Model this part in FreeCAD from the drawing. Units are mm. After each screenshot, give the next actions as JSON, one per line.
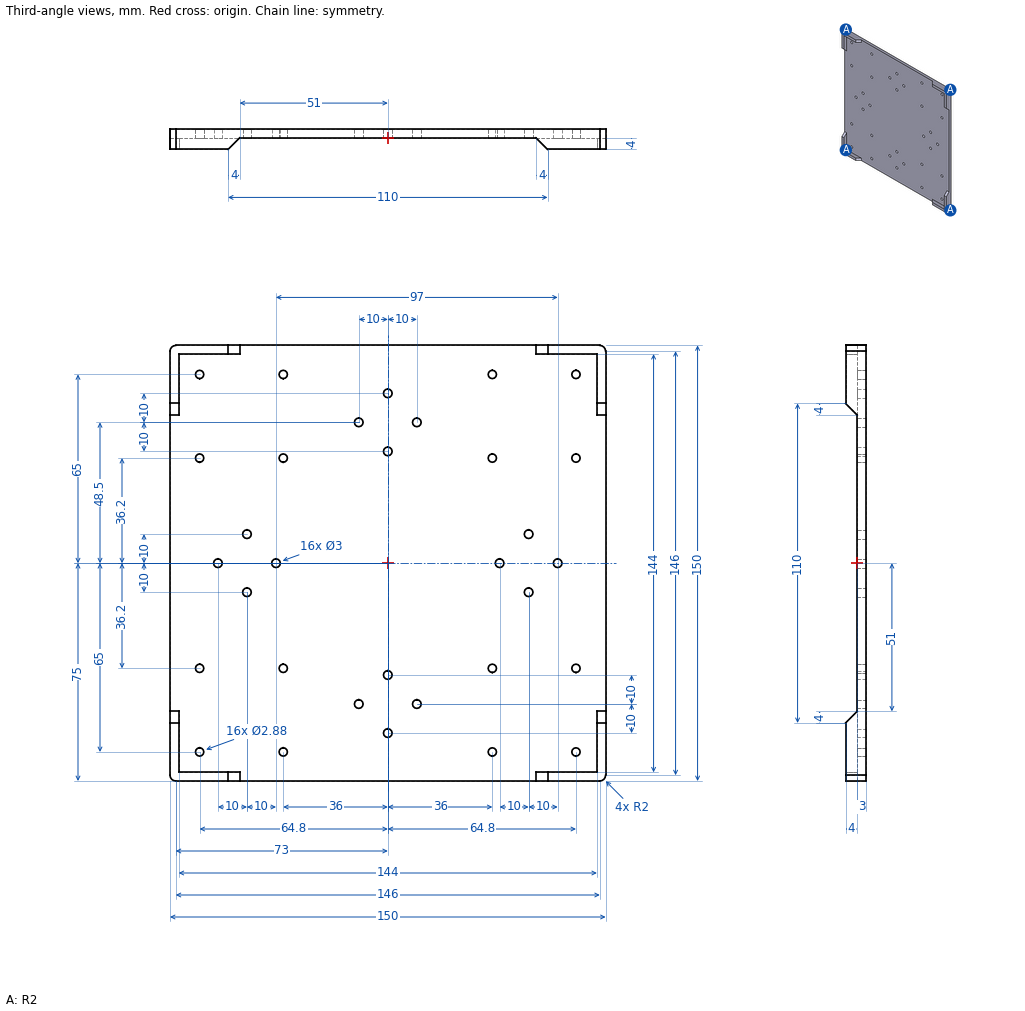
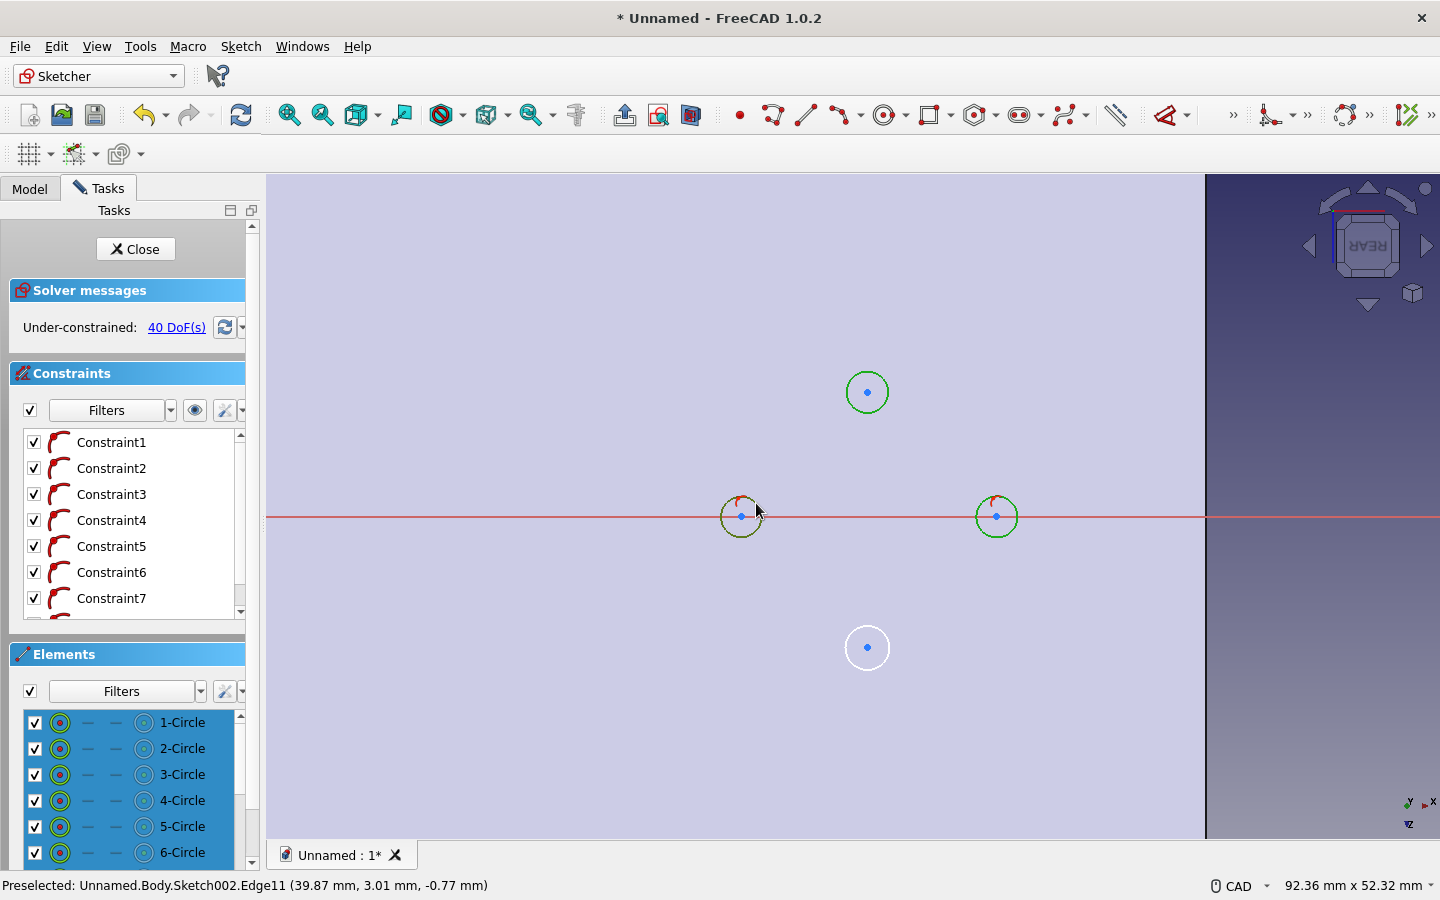
{"action": "scroll", "coordinate": [1014, 502], "scroll_direction": "down", "scroll_amount": 6}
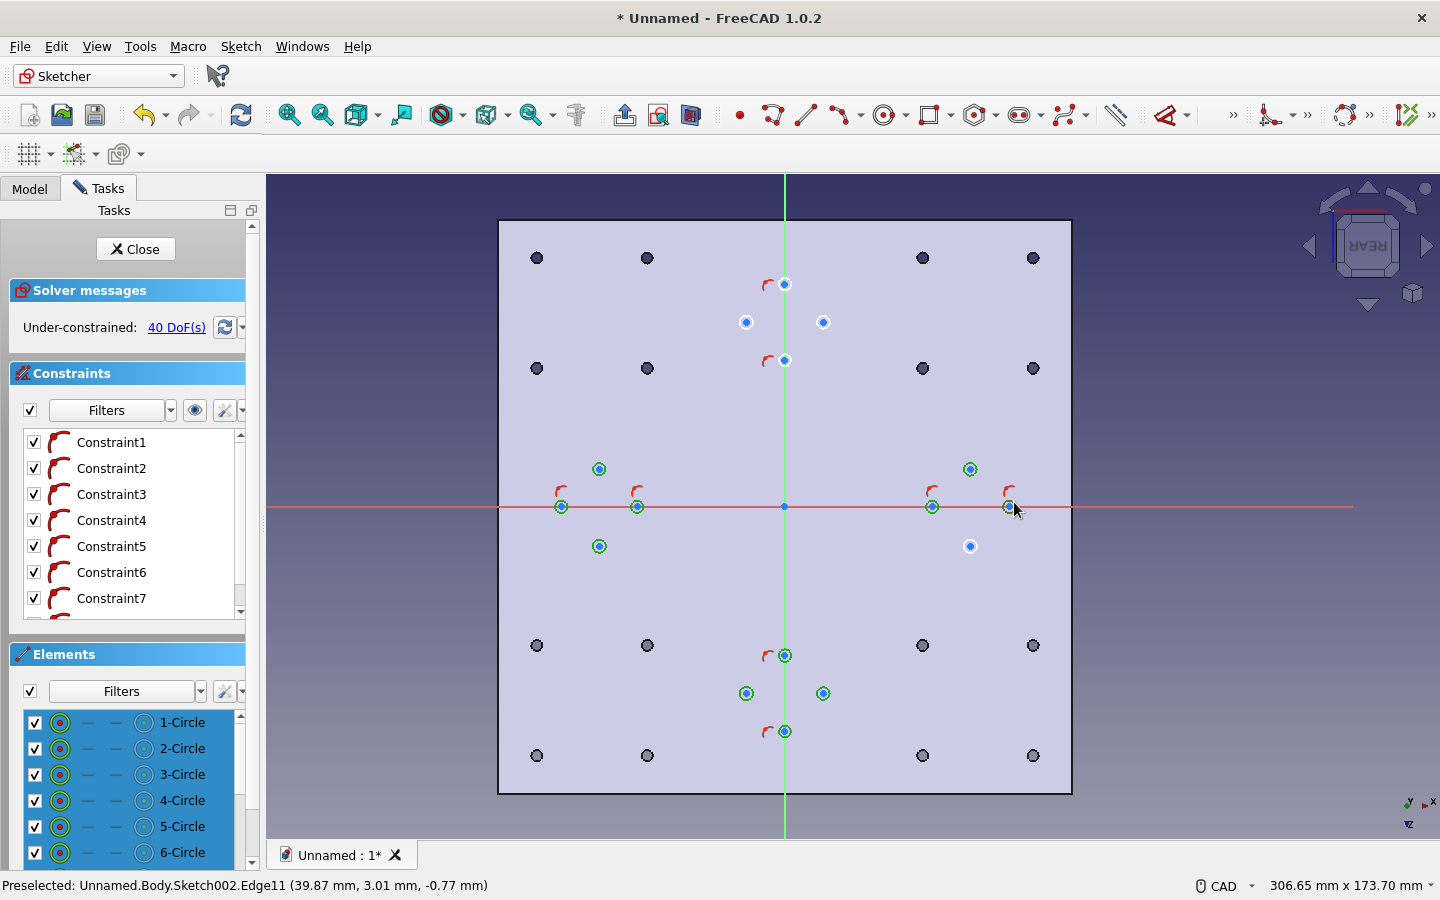
{"action": "scroll", "coordinate": [789, 356], "scroll_direction": "up", "scroll_amount": 7}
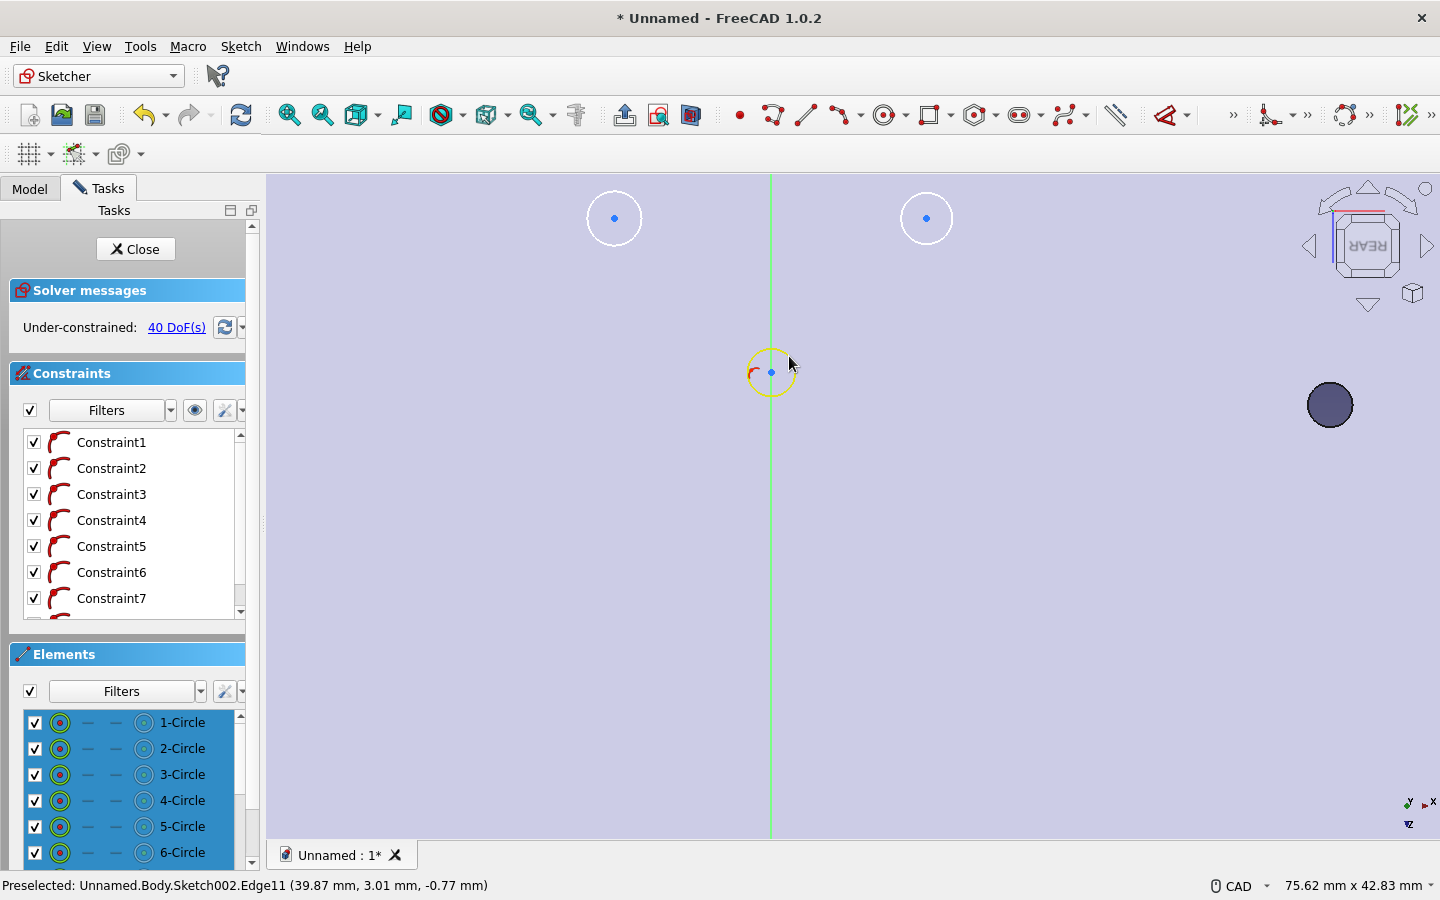
{"action": "left_click", "coordinate": [788, 356]}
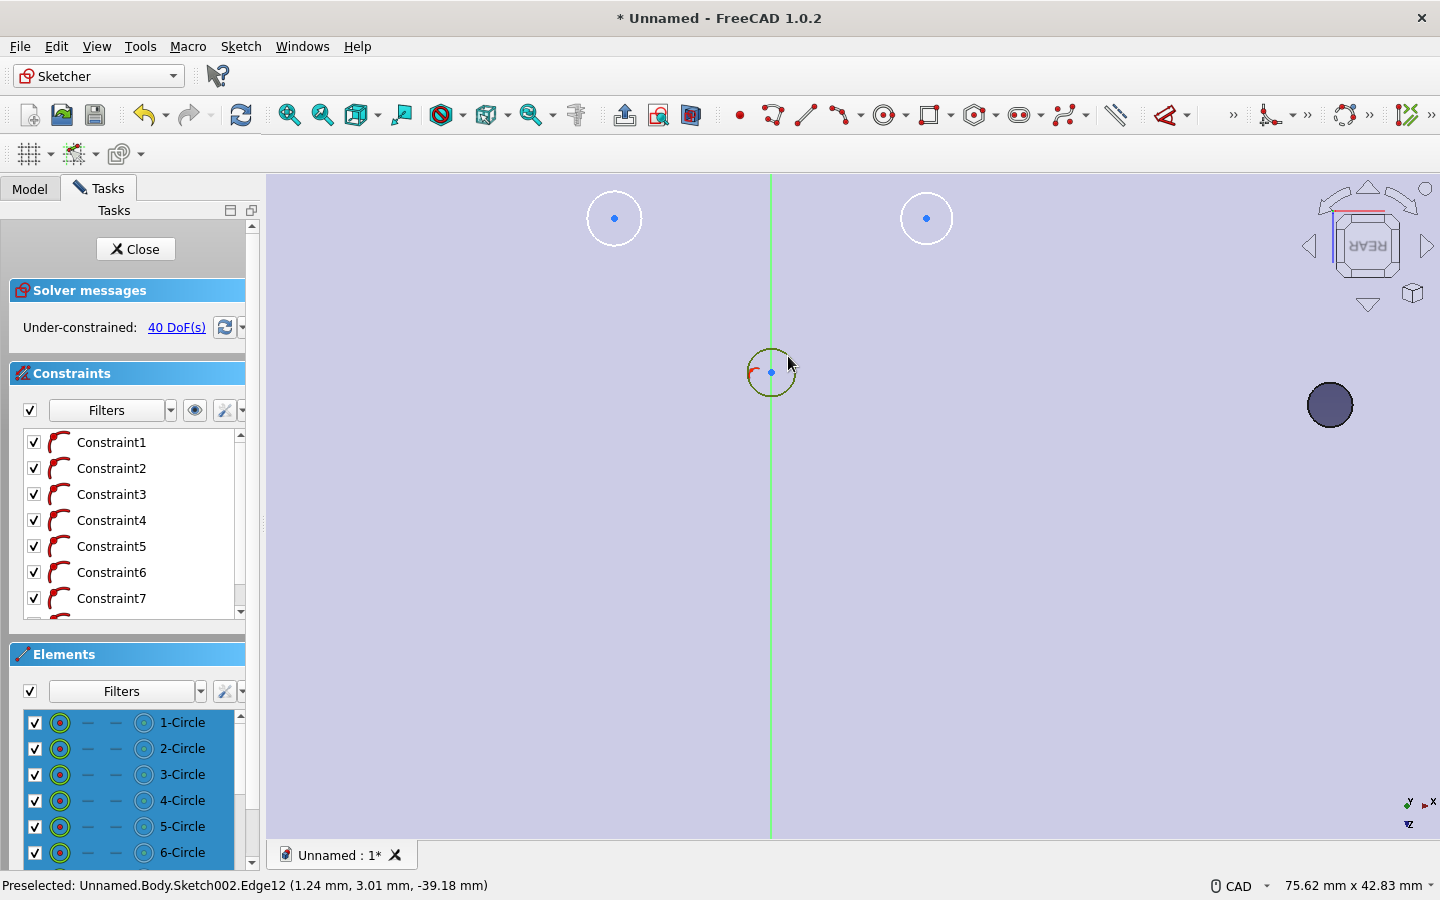
{"action": "left_click", "coordinate": [909, 237]}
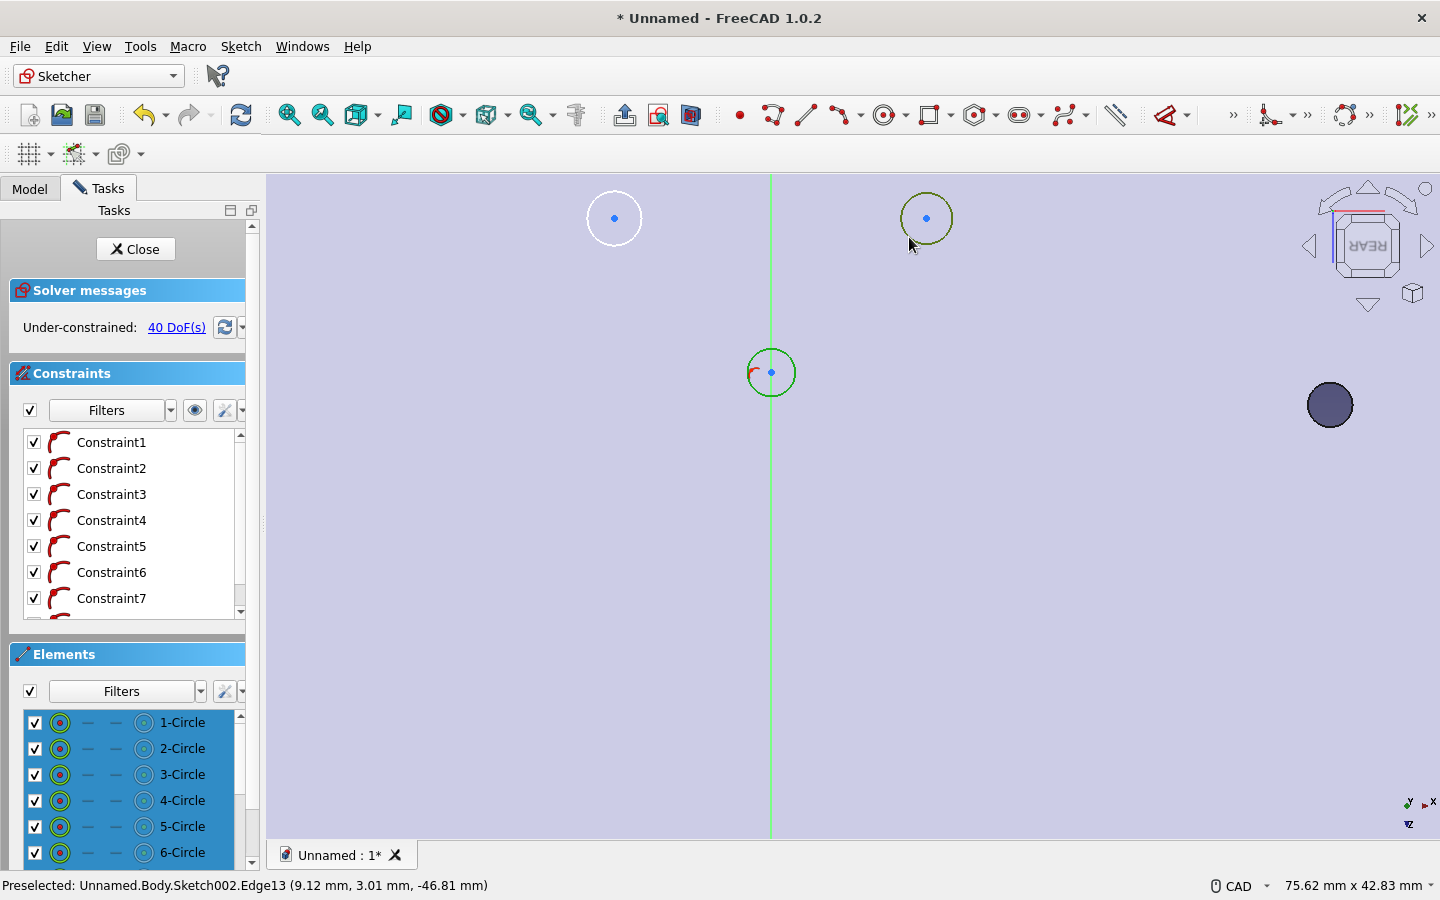
{"action": "scroll", "coordinate": [789, 356], "scroll_direction": "down", "scroll_amount": 7}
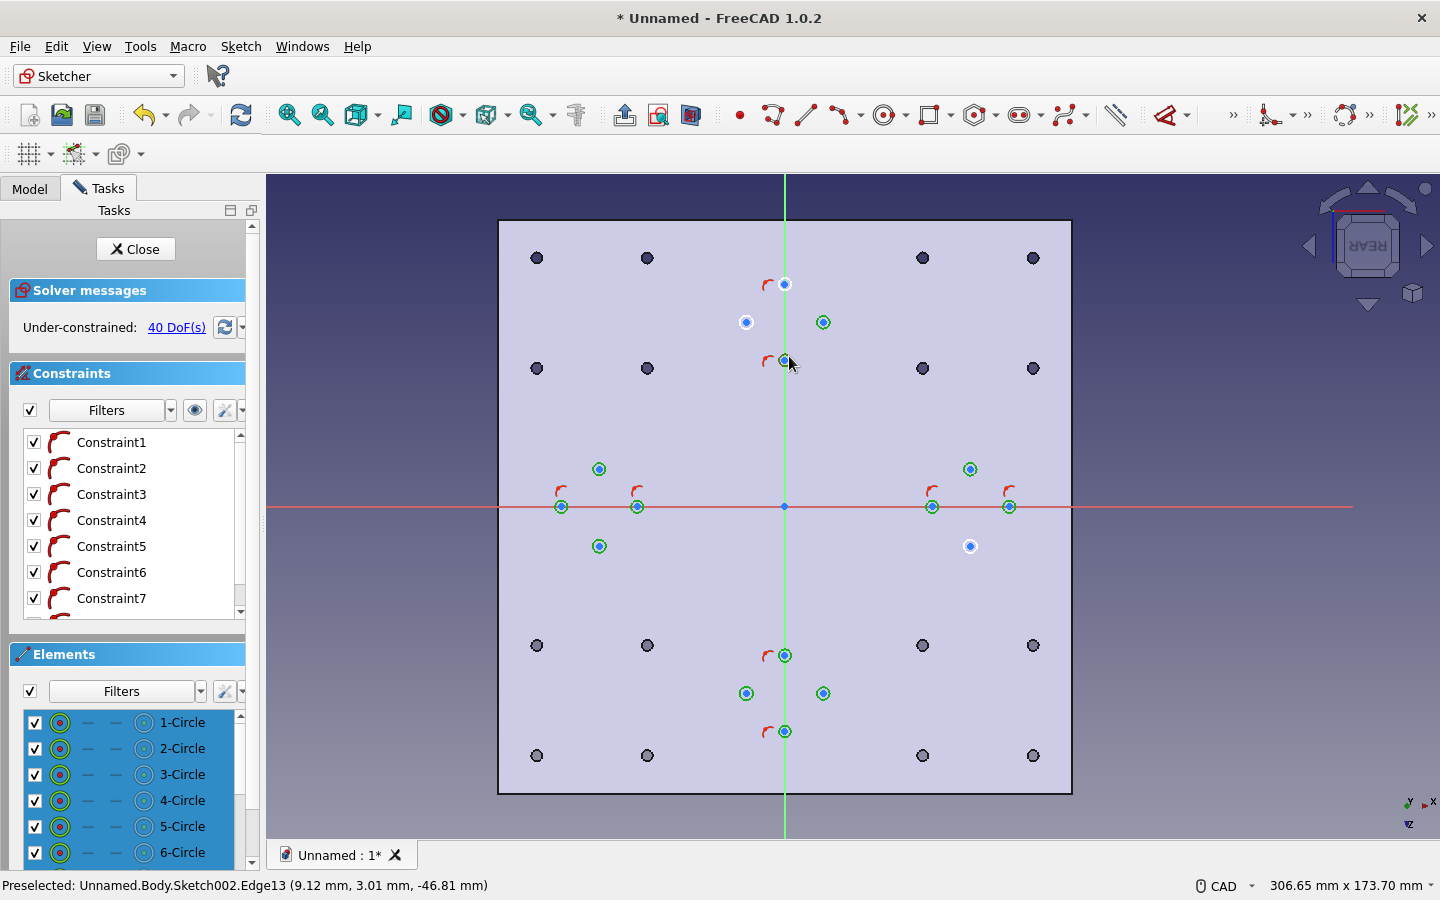
{"action": "scroll", "coordinate": [789, 280], "scroll_direction": "up", "scroll_amount": 6}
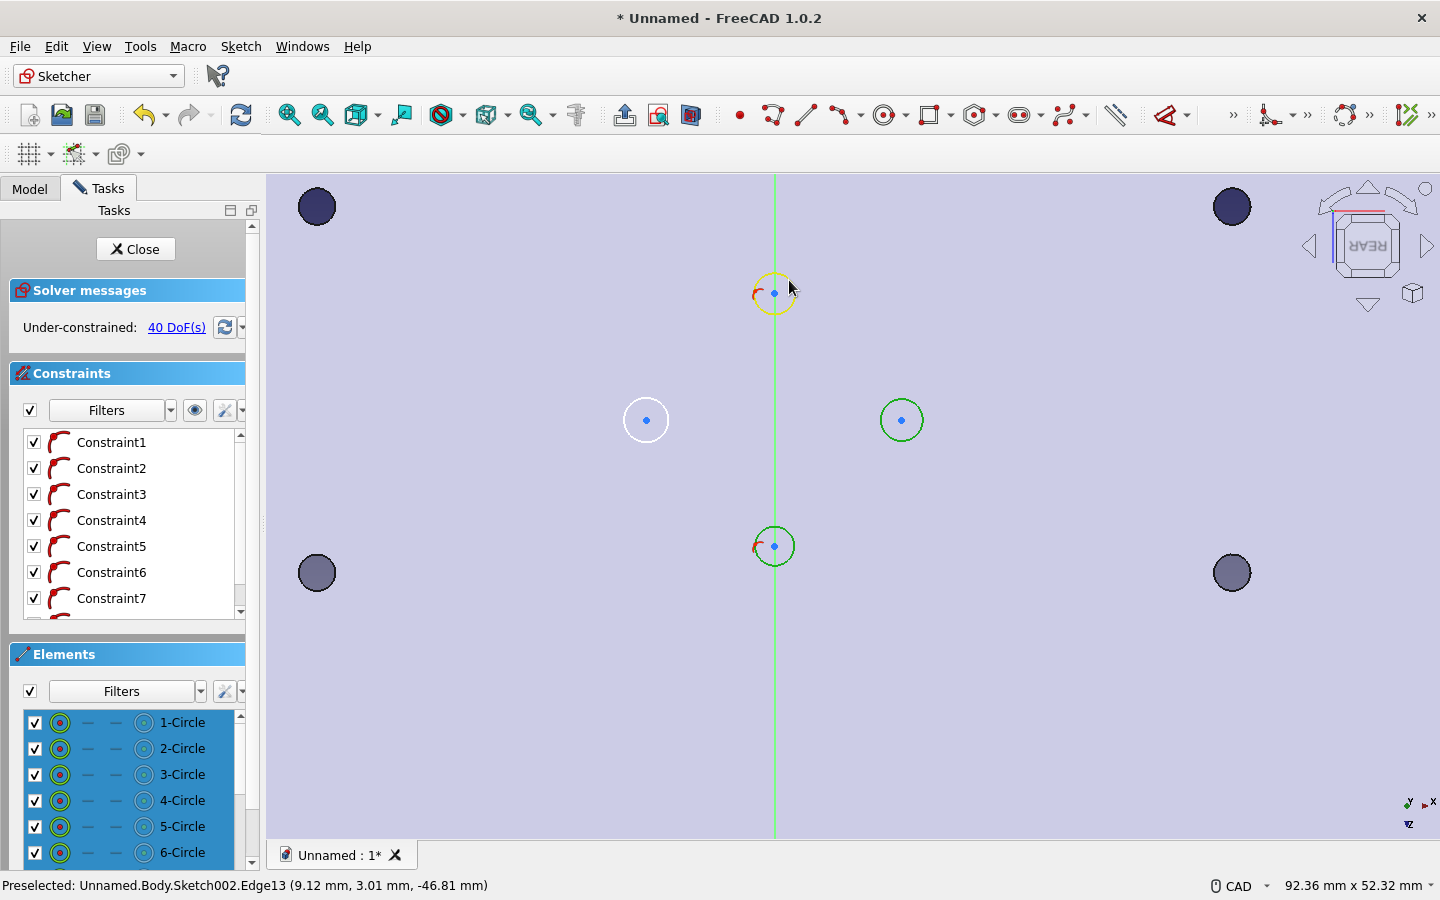
{"action": "left_click", "coordinate": [789, 279]}